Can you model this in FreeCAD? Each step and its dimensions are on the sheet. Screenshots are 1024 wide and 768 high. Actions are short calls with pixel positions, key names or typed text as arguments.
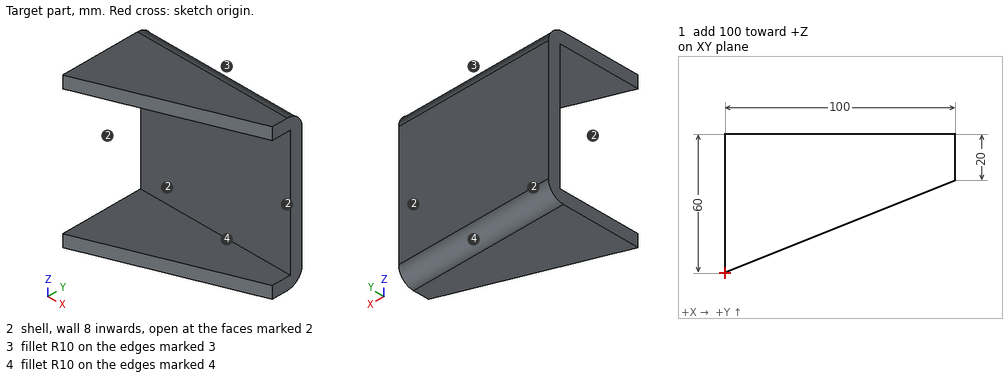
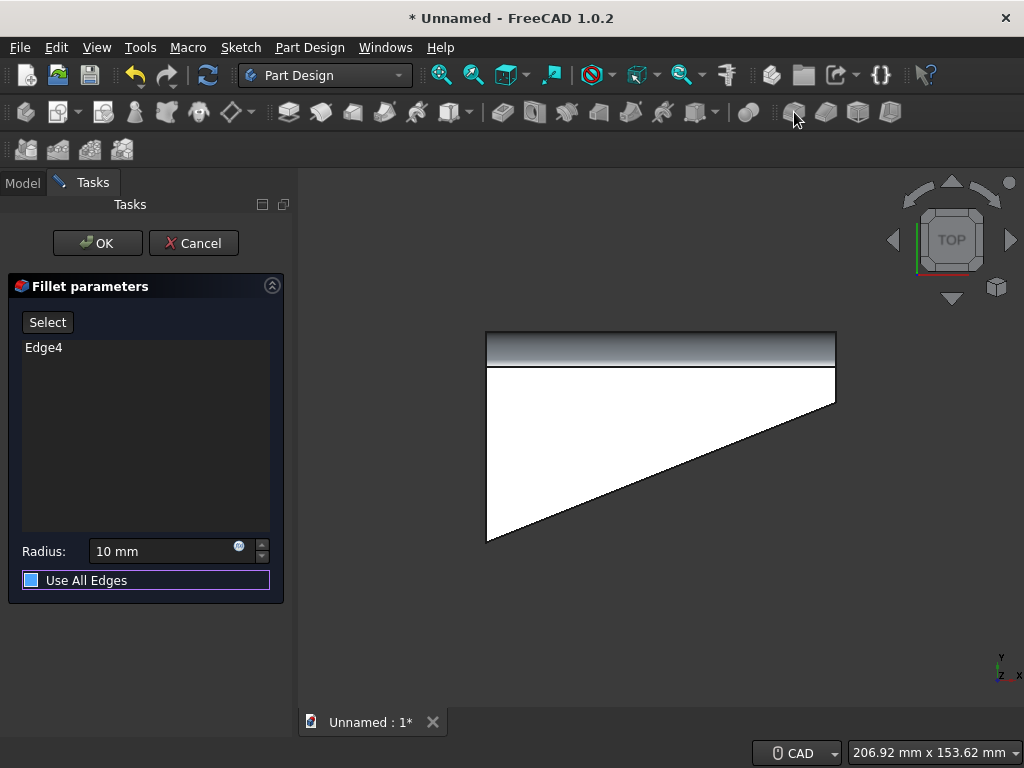
click(98, 243)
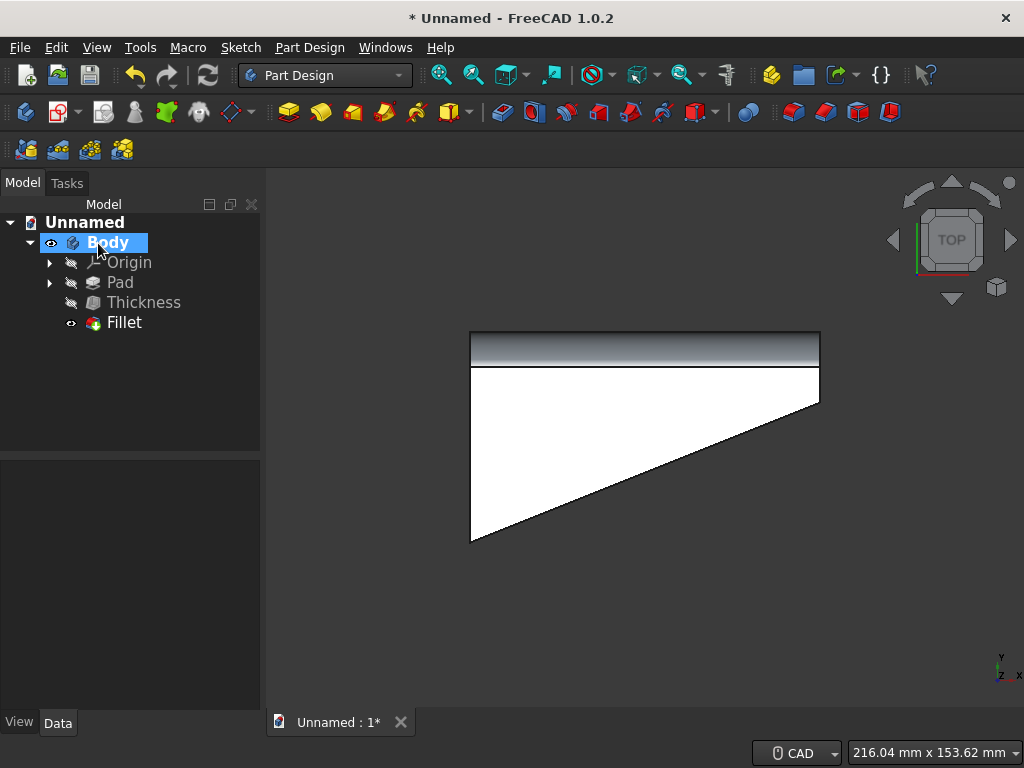
key(0)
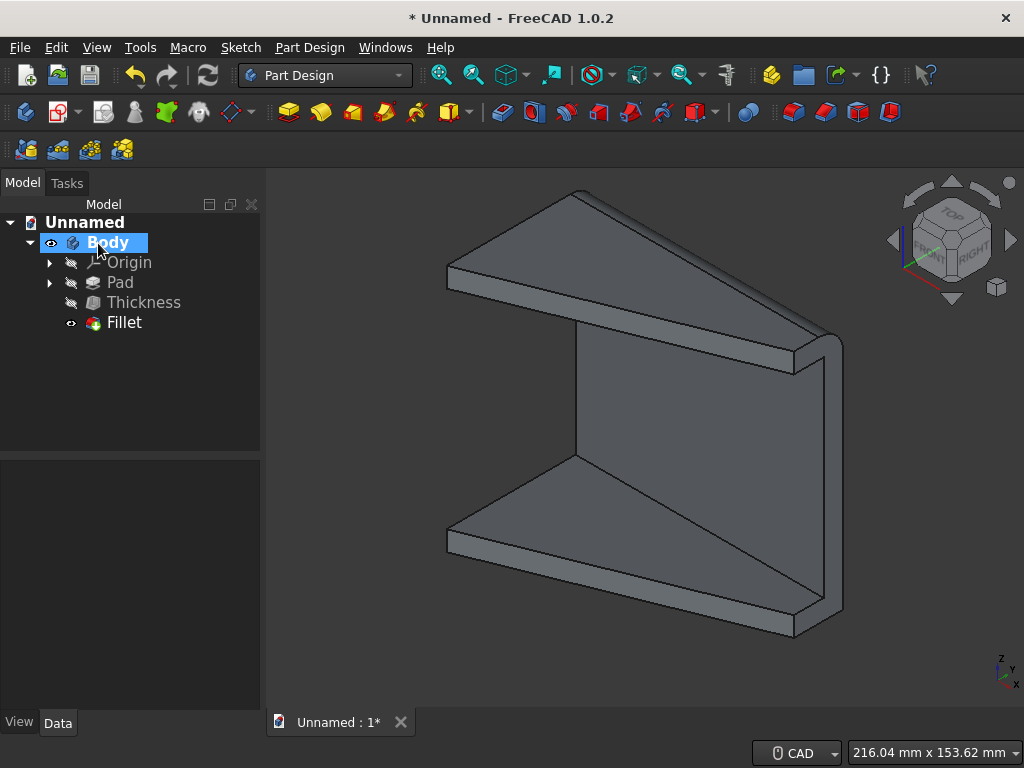
key(2)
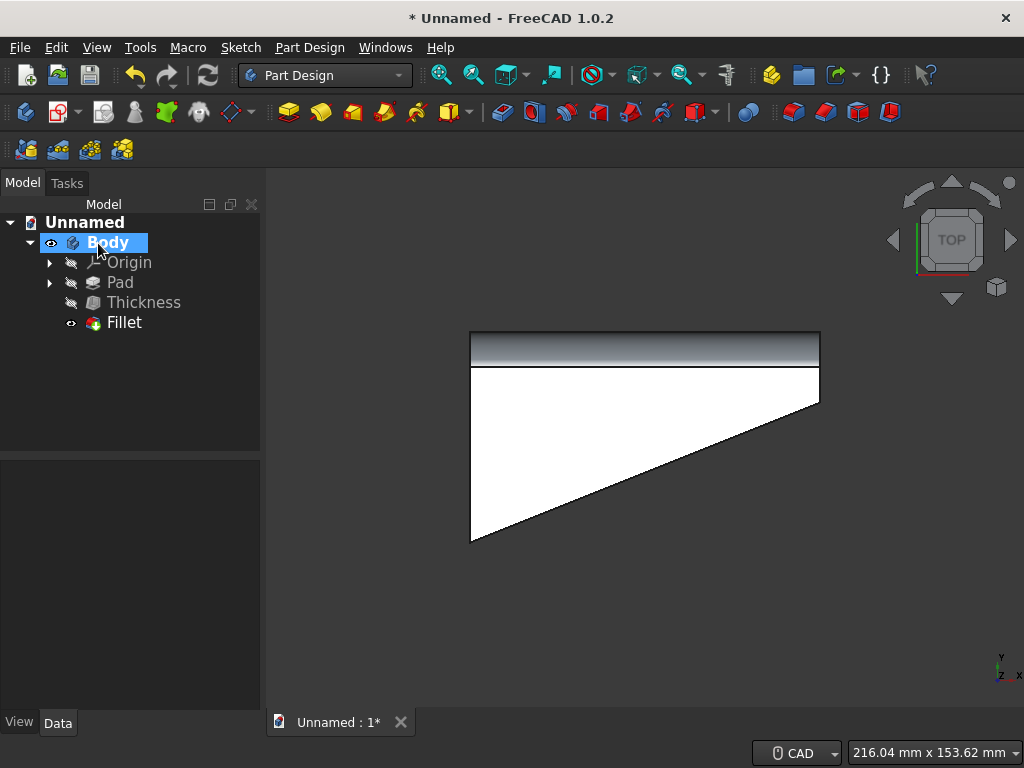
key(1)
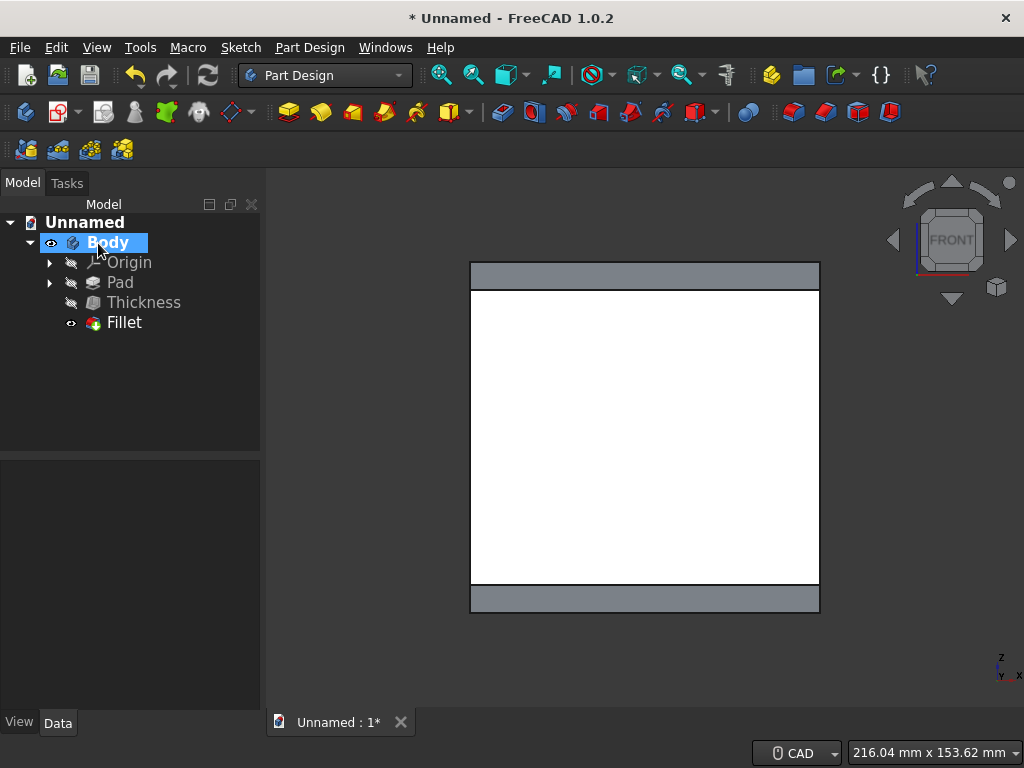
key(3)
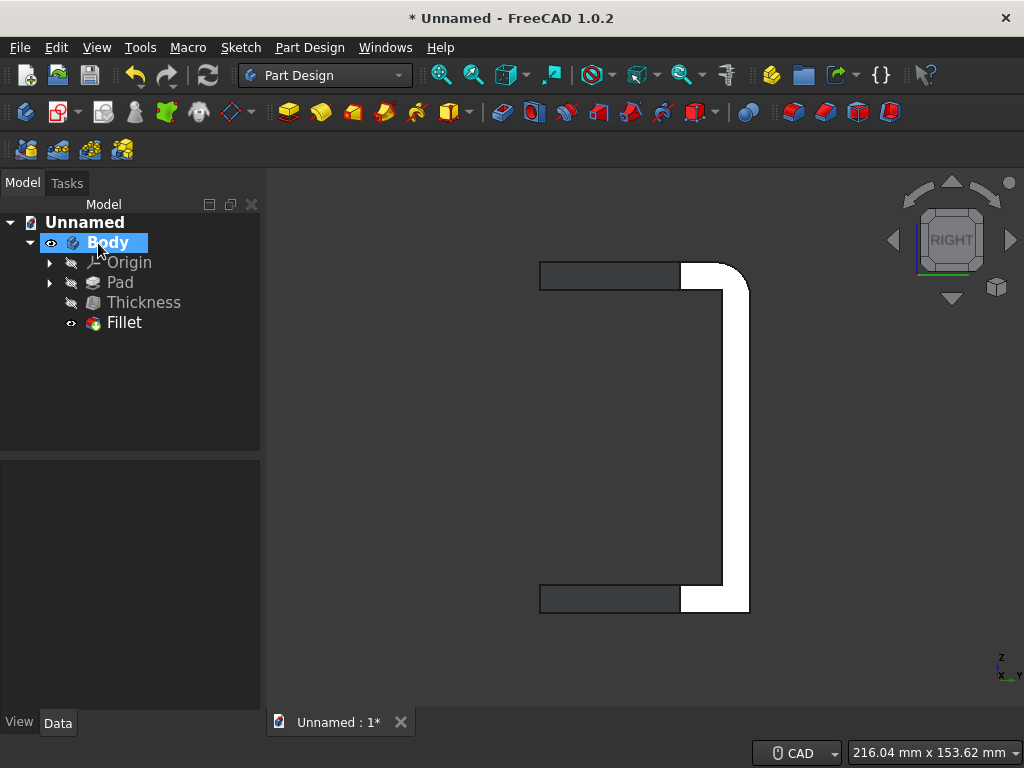
key(5)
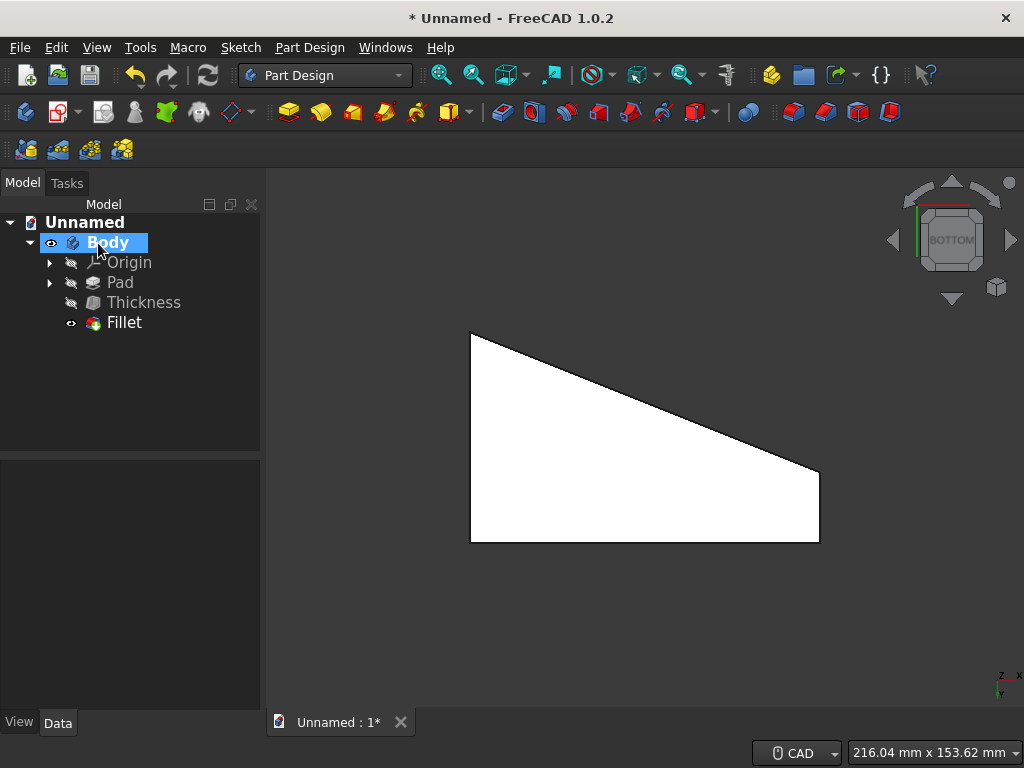
click(645, 542)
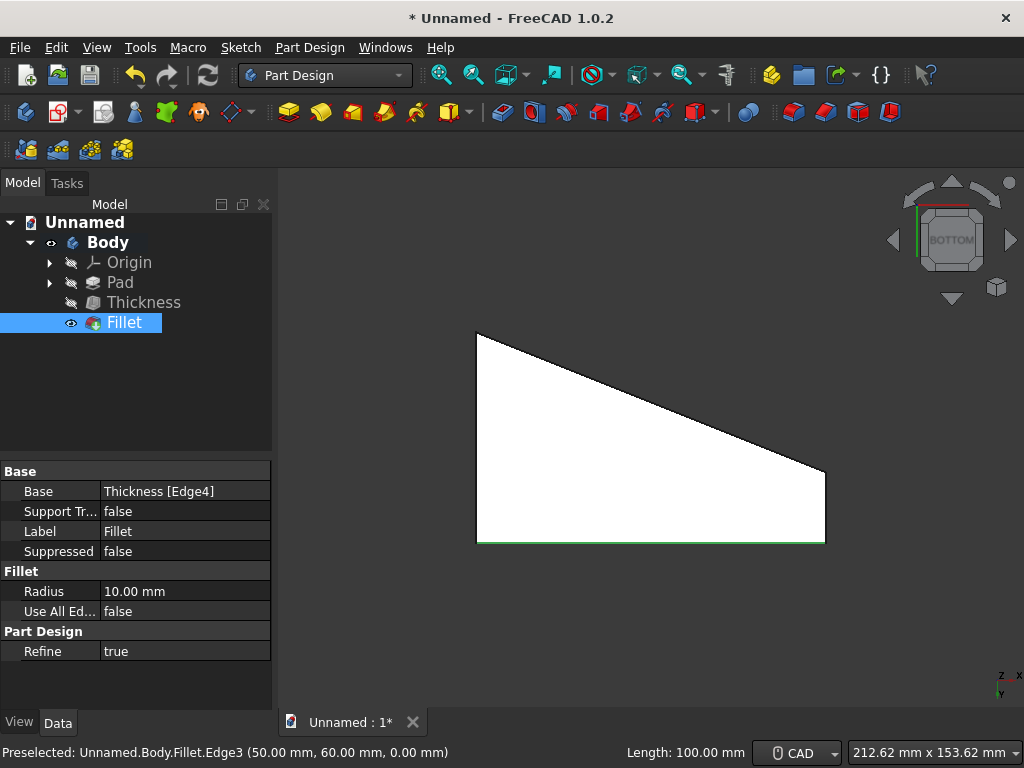
click(794, 112)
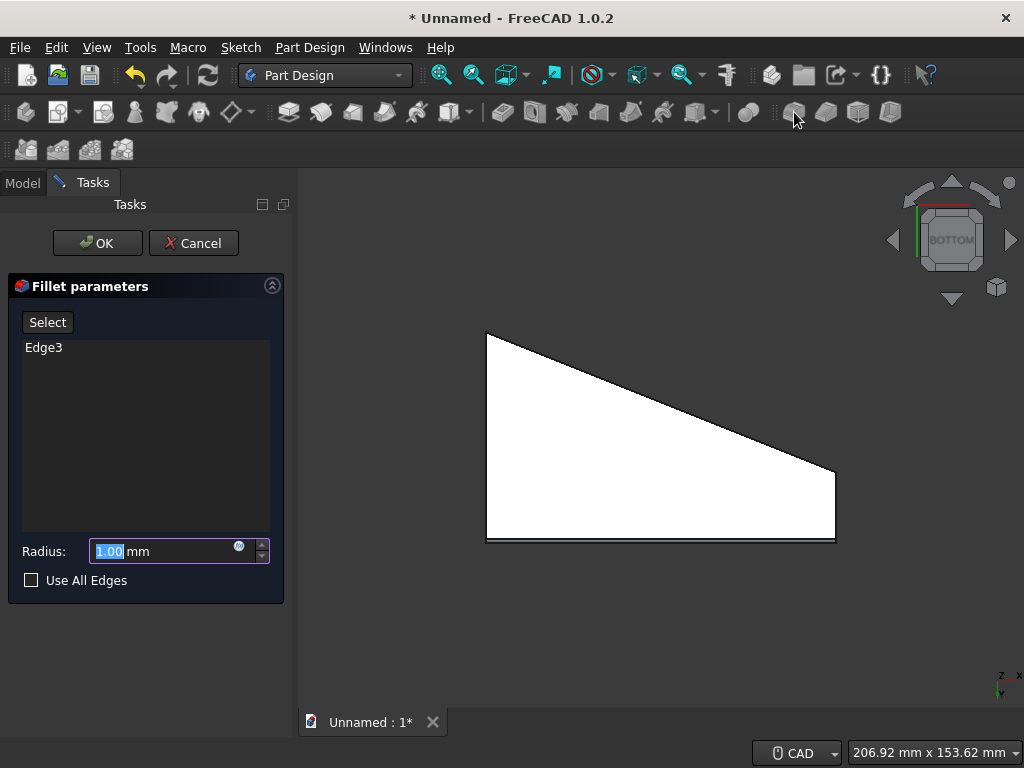
text(10)
key(Tab)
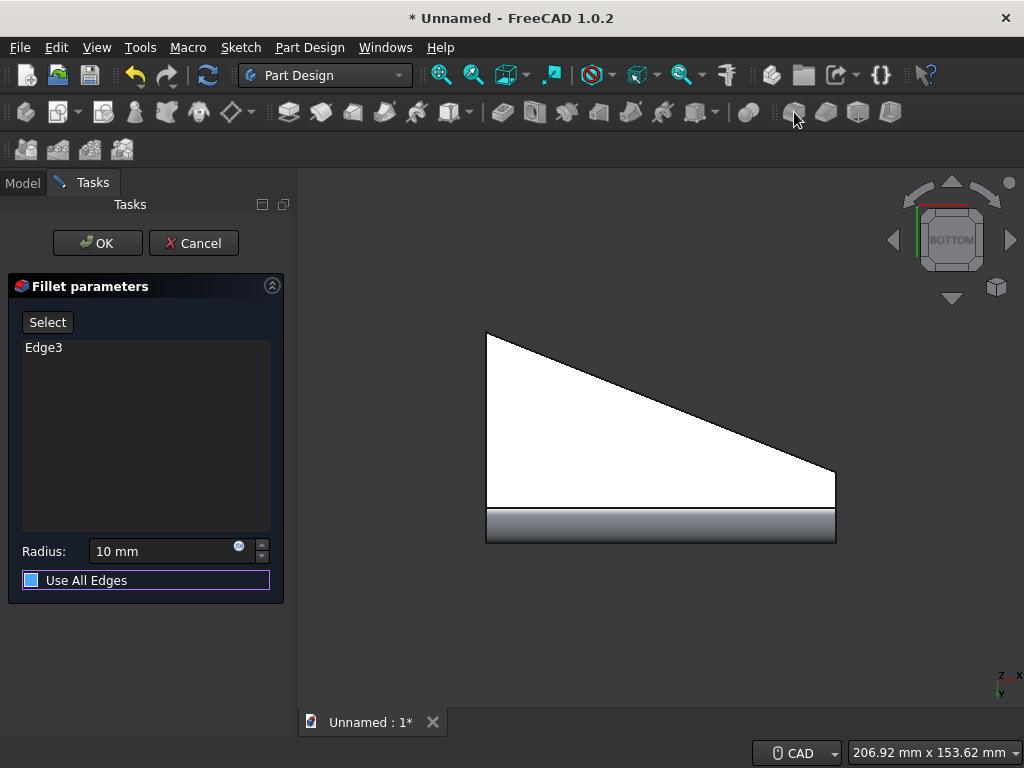
click(98, 243)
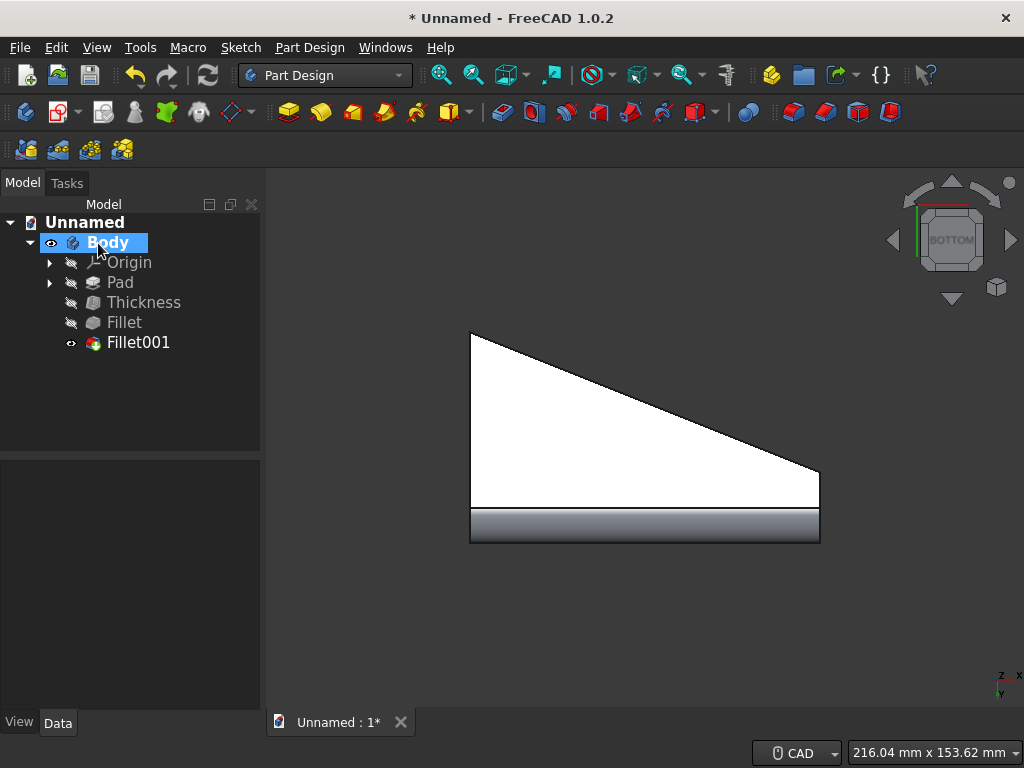
key(0)